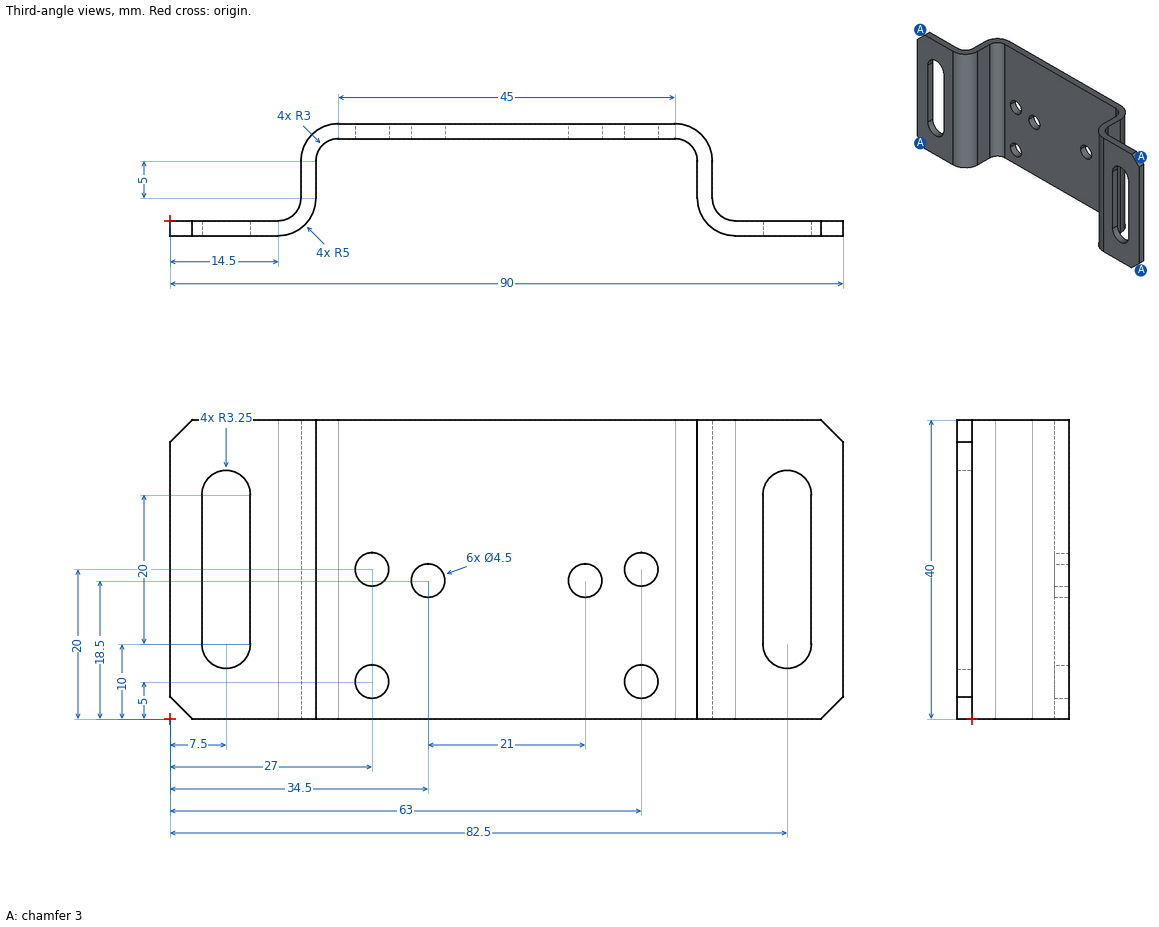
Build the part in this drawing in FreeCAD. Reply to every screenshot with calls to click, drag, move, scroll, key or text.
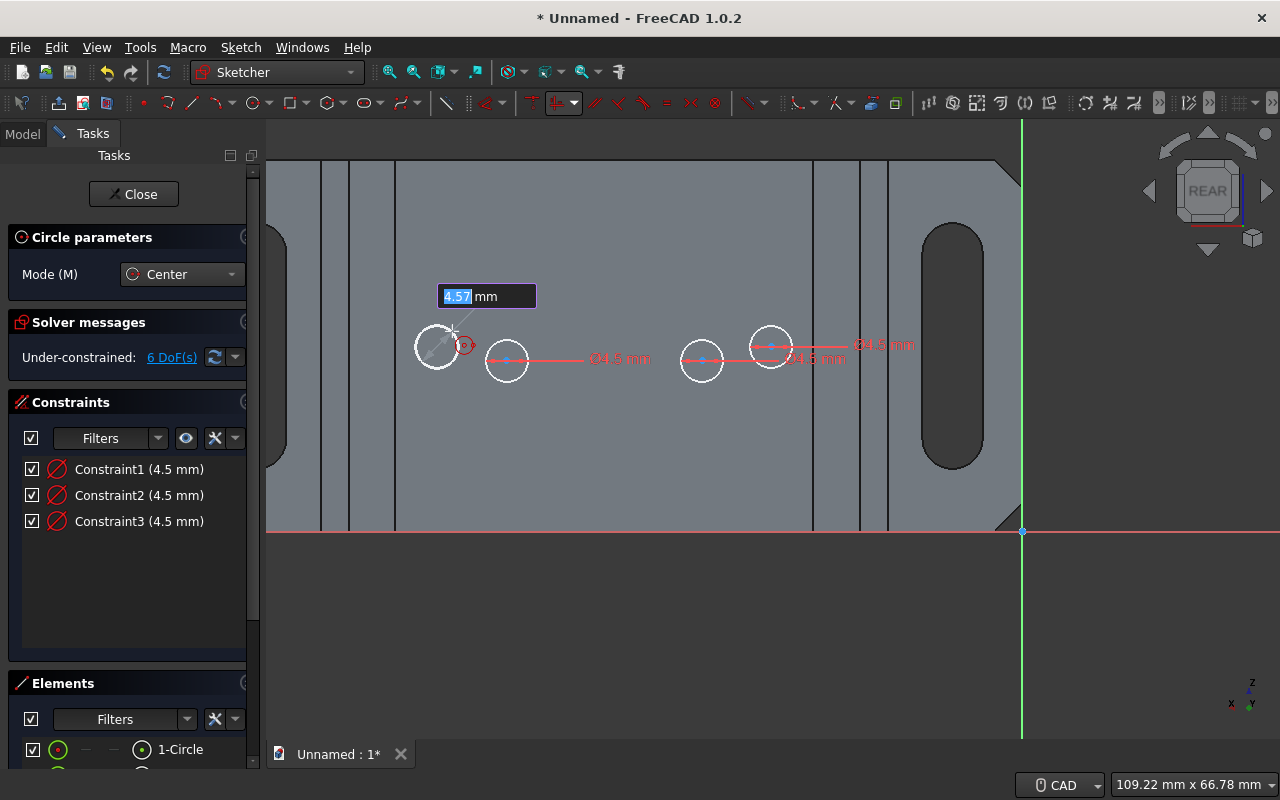
text(4.5)
key(Return)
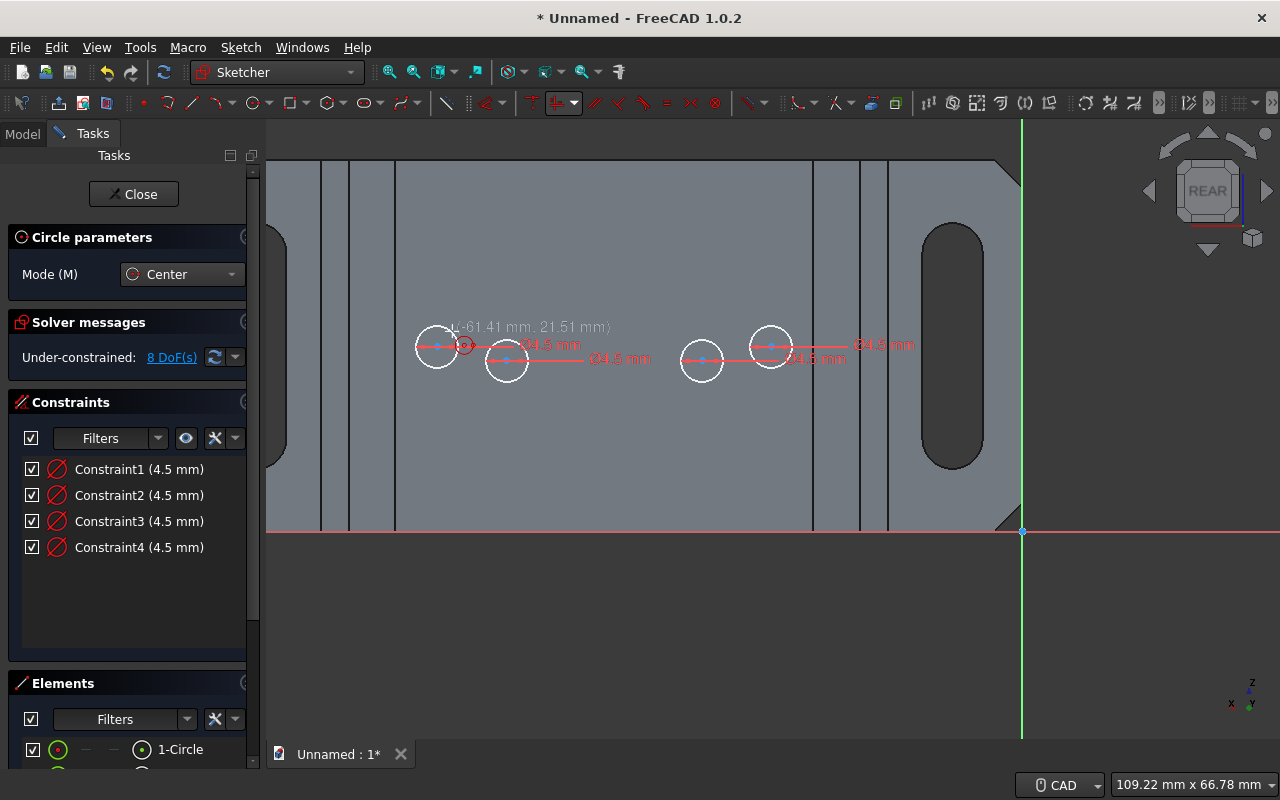
click(771, 485)
move(786, 470)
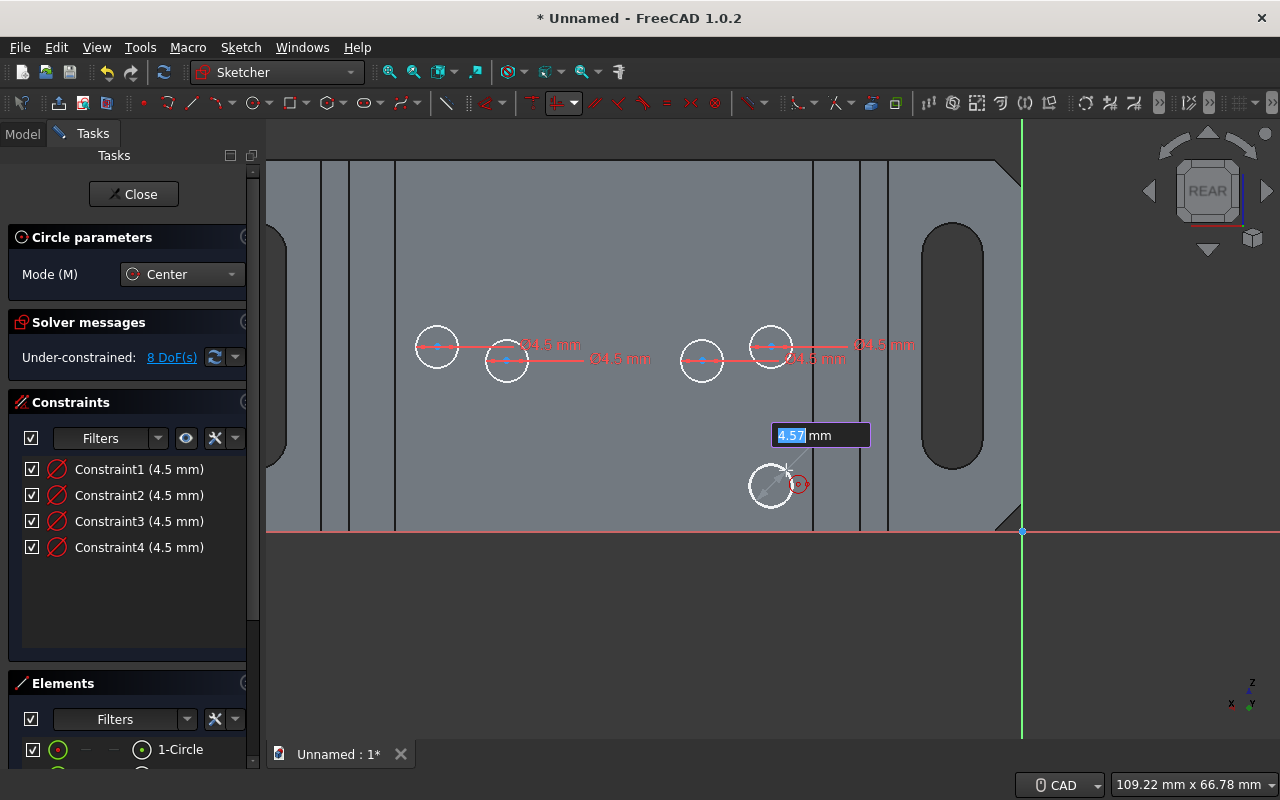
text(4.5)
key(Return)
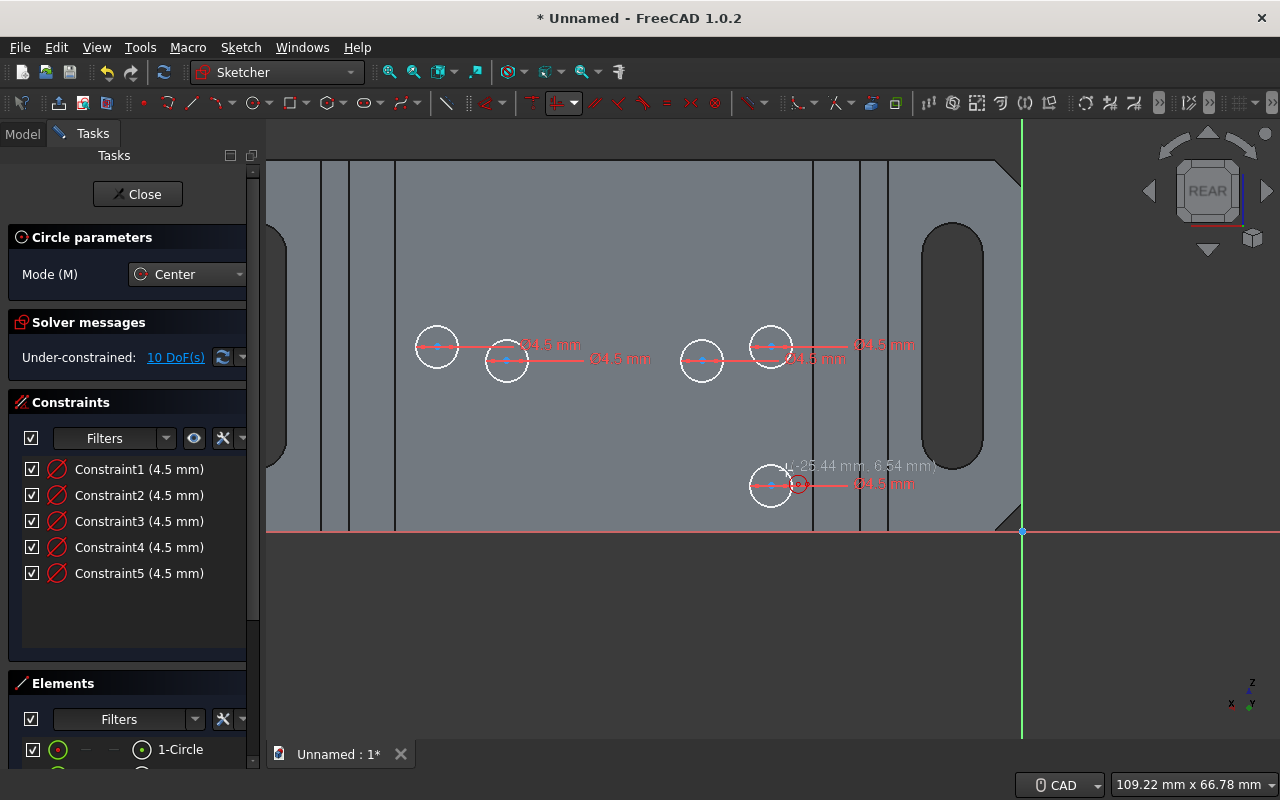
click(437, 485)
move(452, 470)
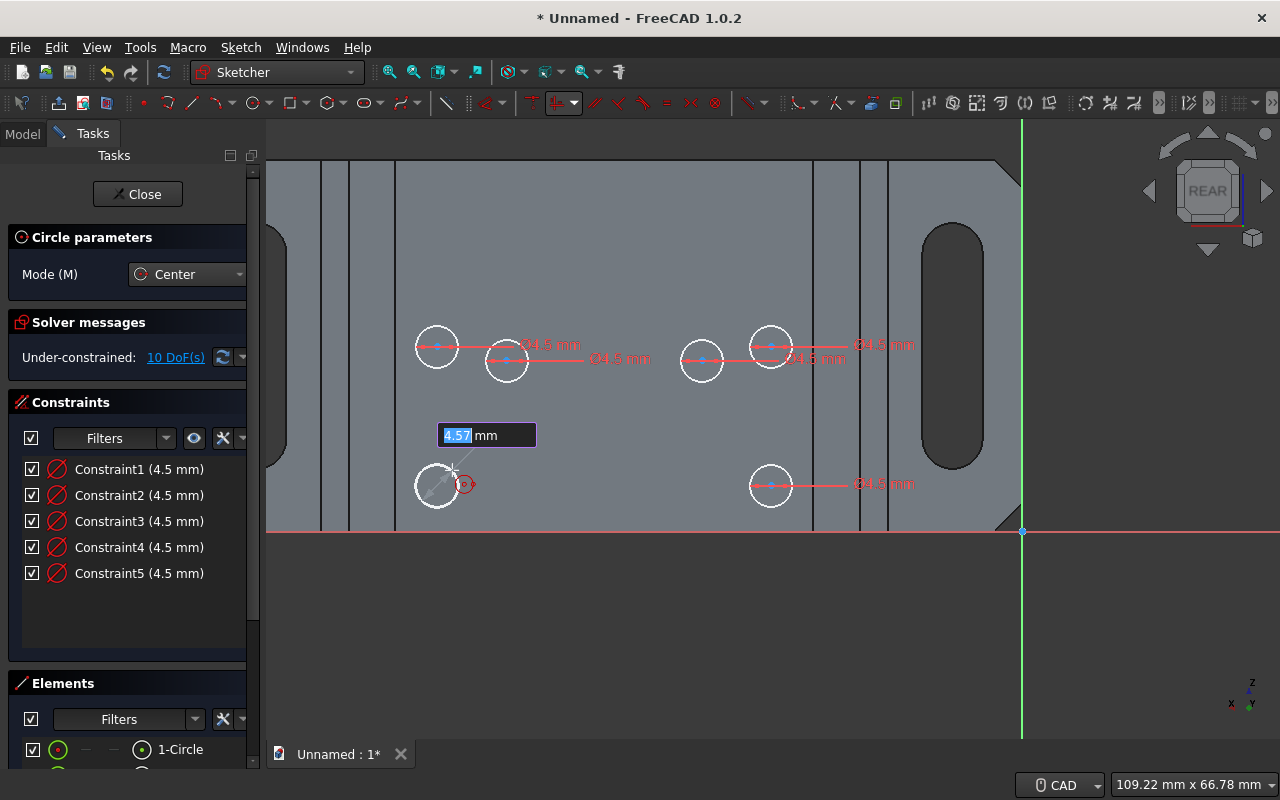
text(4.5)
key(Return)
key(Escape)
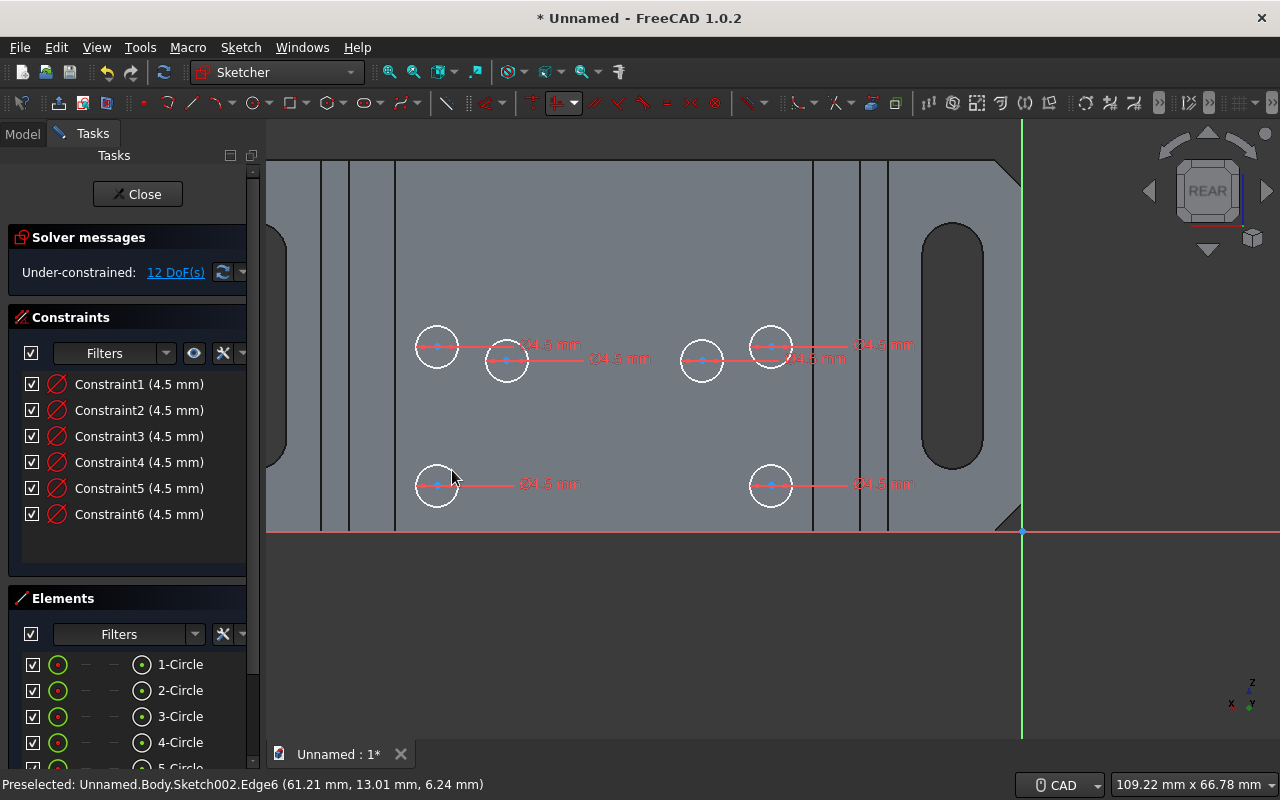
key(d)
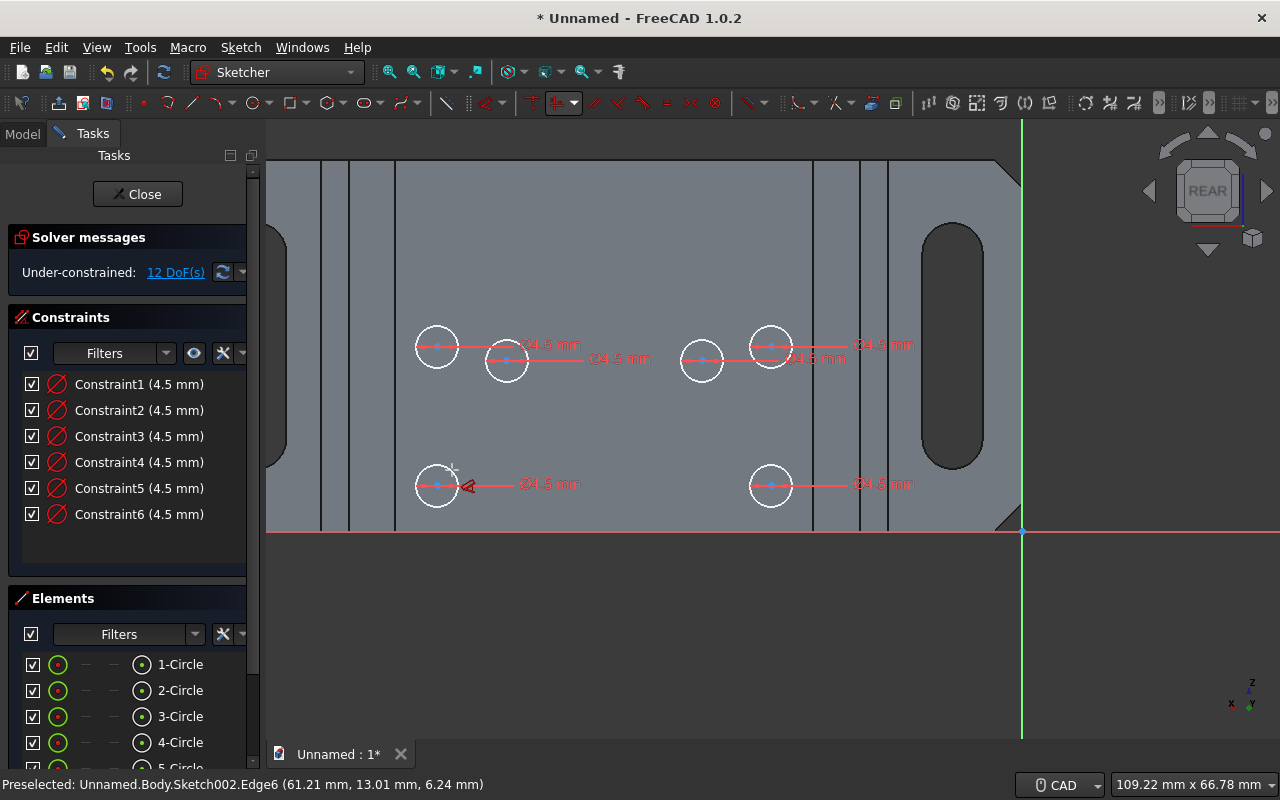
click(771, 486)
click(1056, 509)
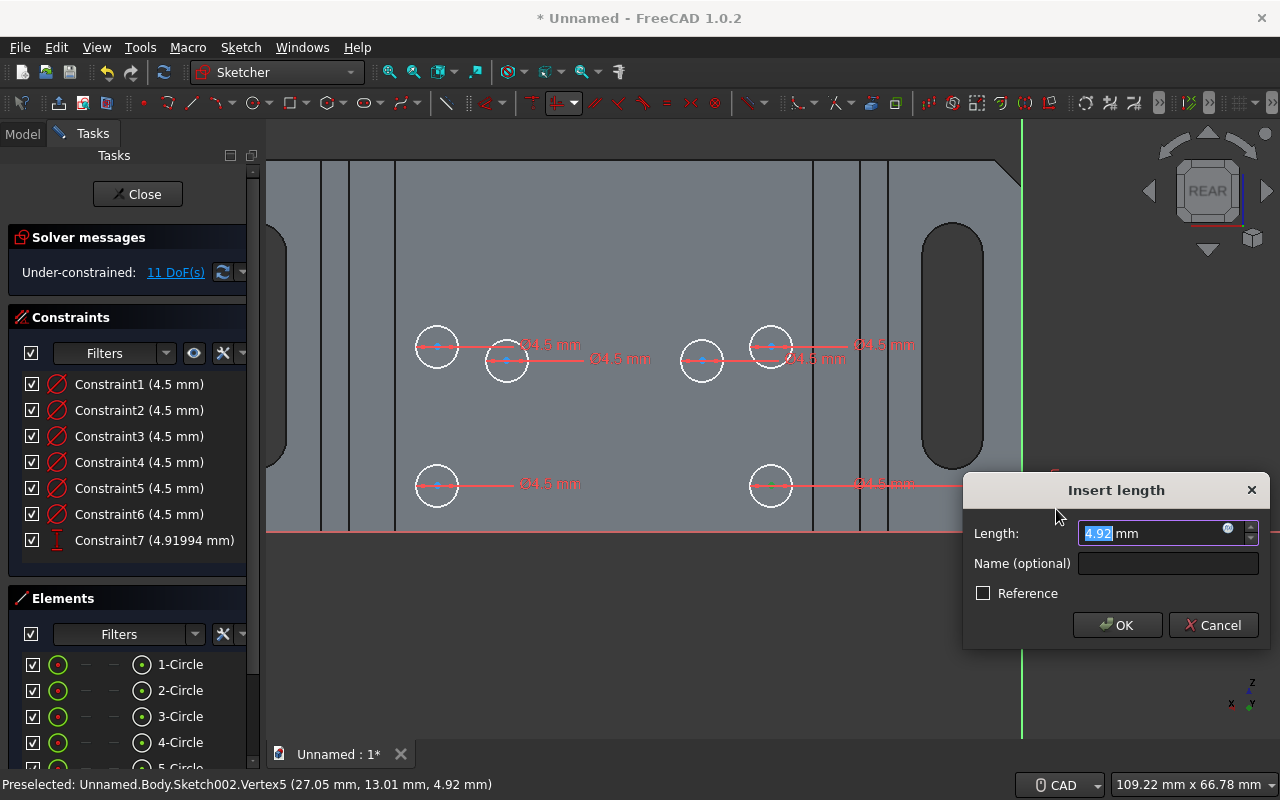
text(5)
key(Return)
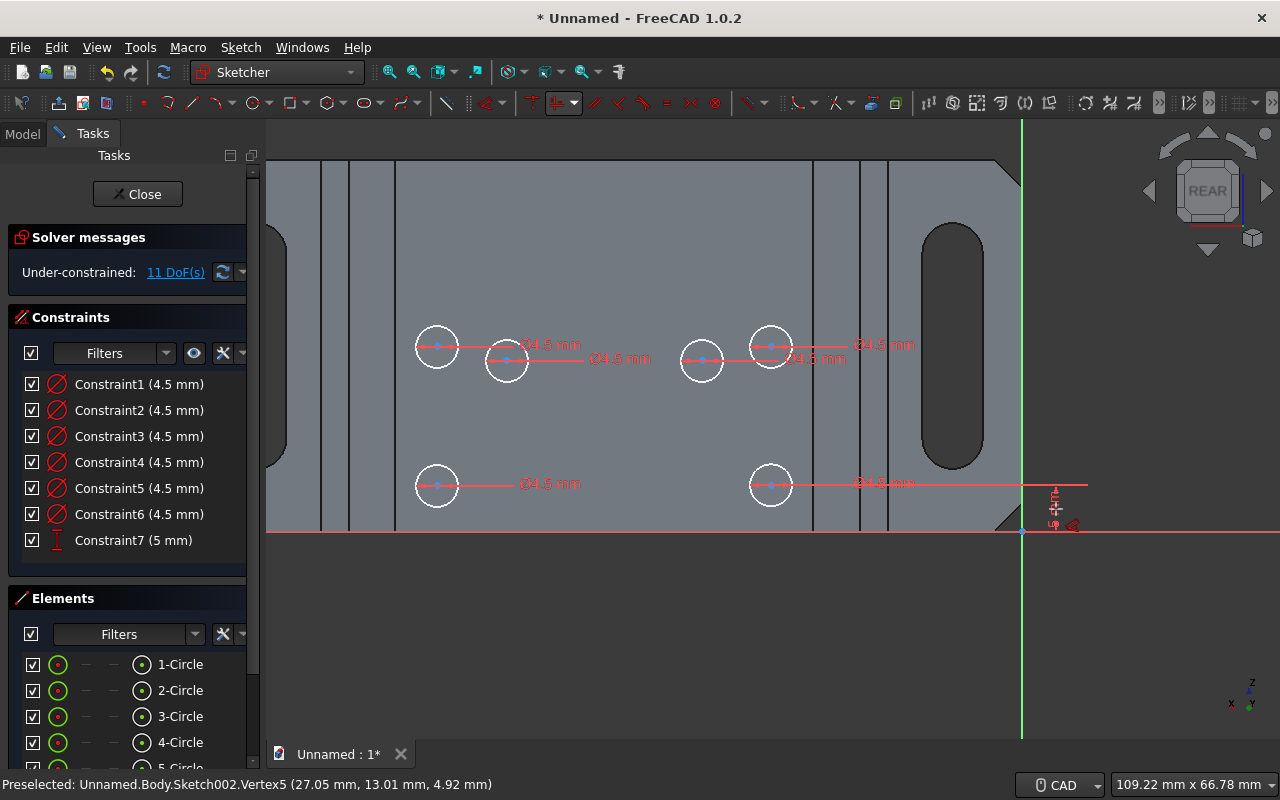
click(437, 486)
click(403, 509)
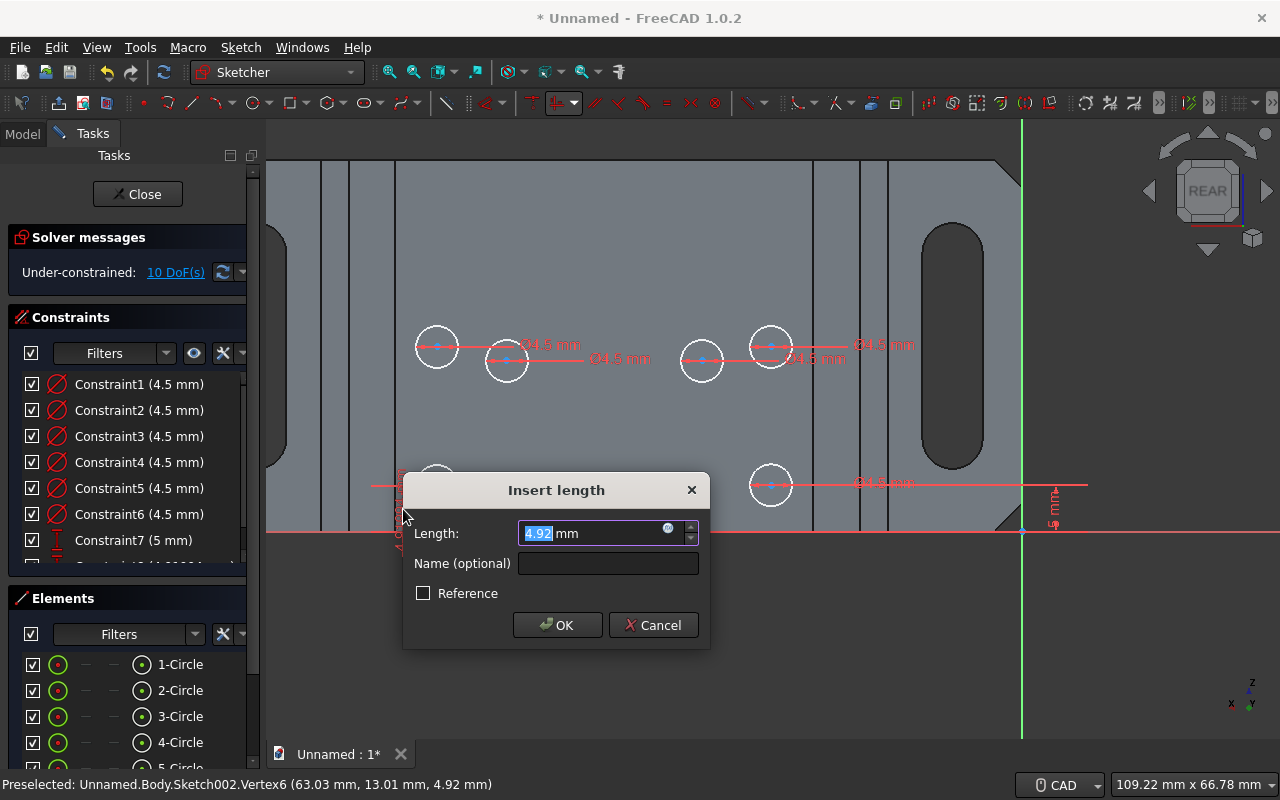
text(5)
key(Return)